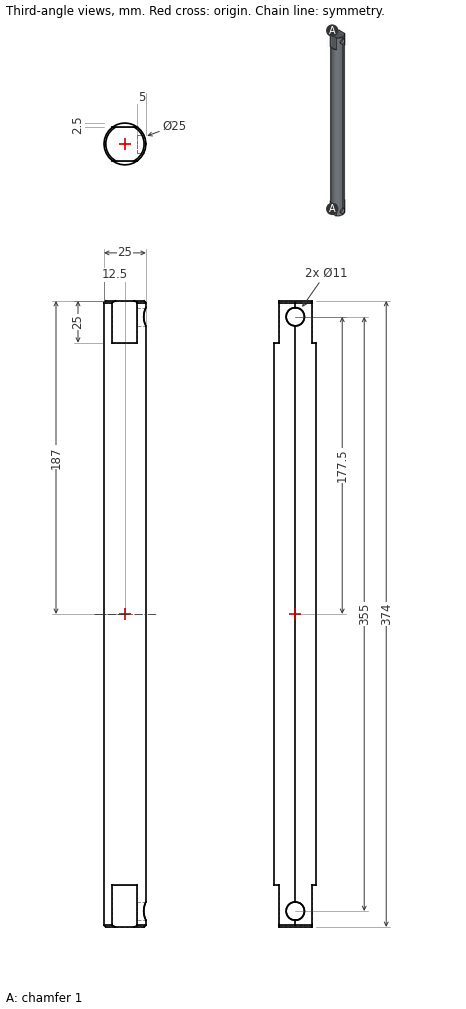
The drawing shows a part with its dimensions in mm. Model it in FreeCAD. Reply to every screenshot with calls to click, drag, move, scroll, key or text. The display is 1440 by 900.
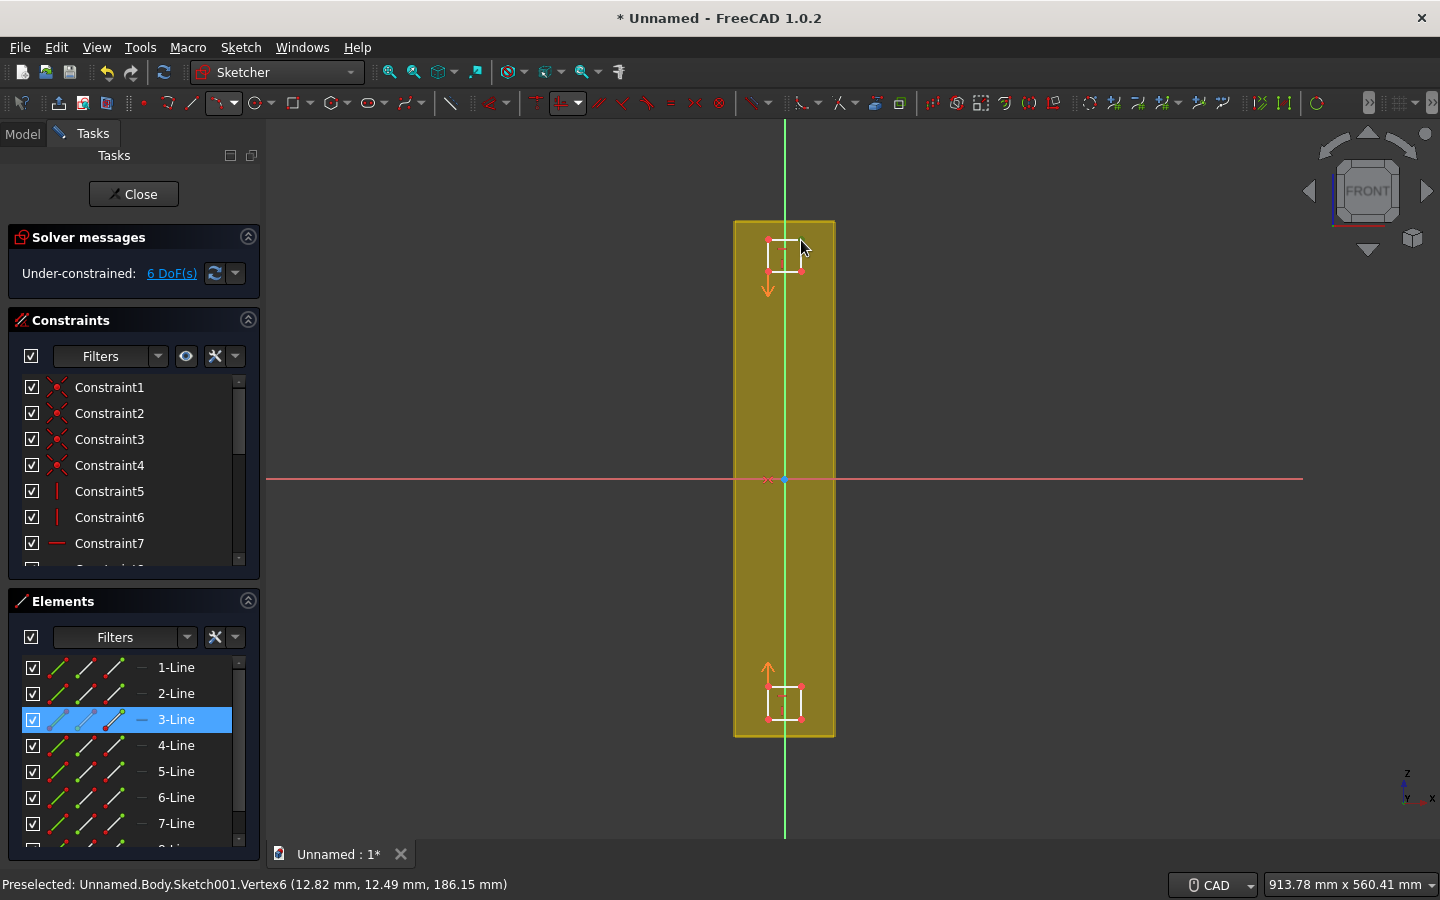
click(801, 720)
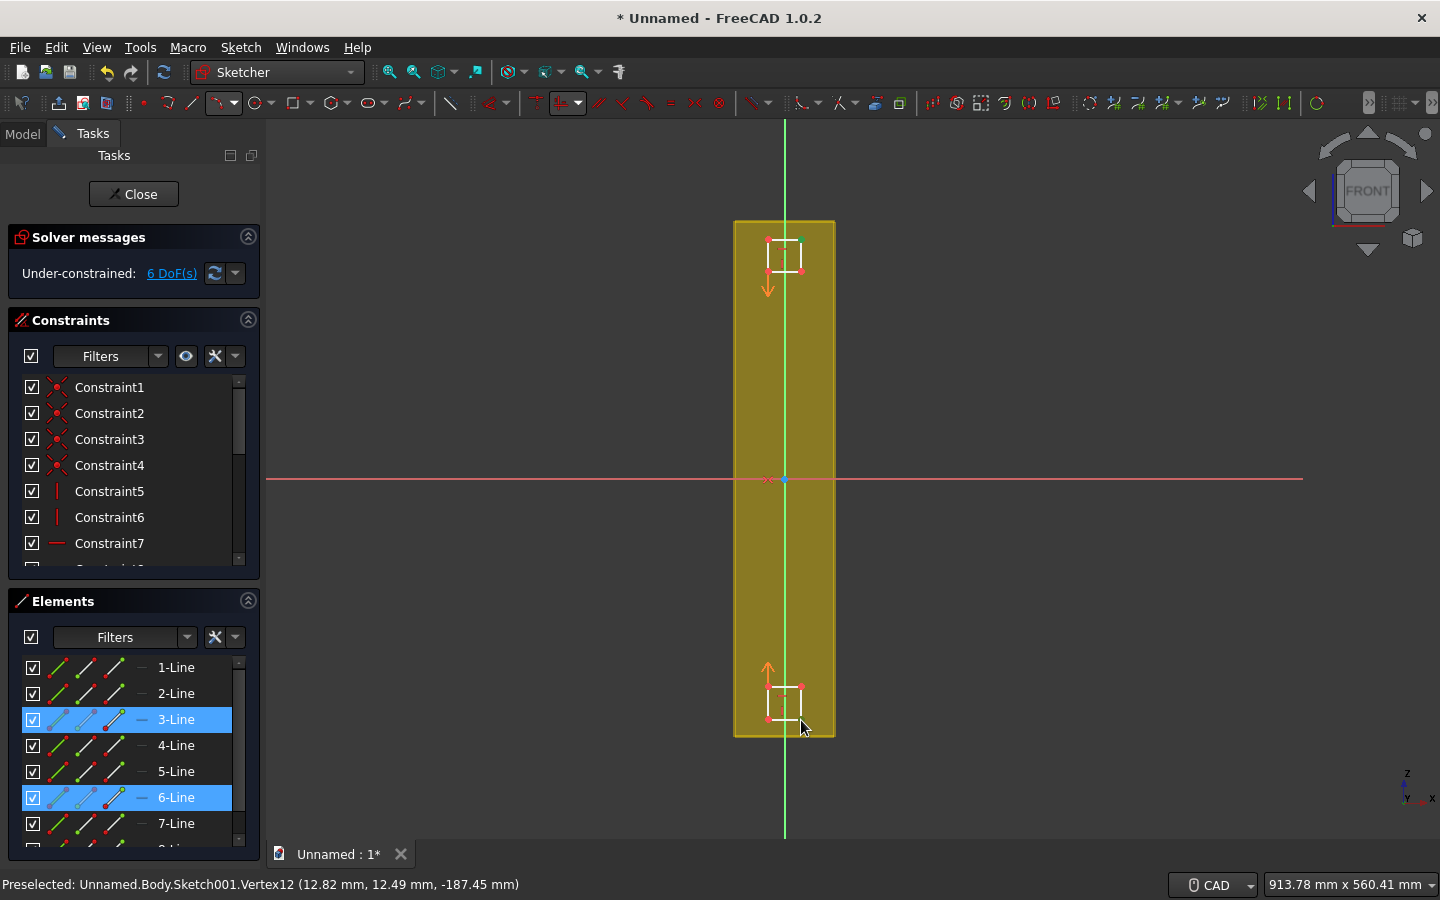
click(364, 479)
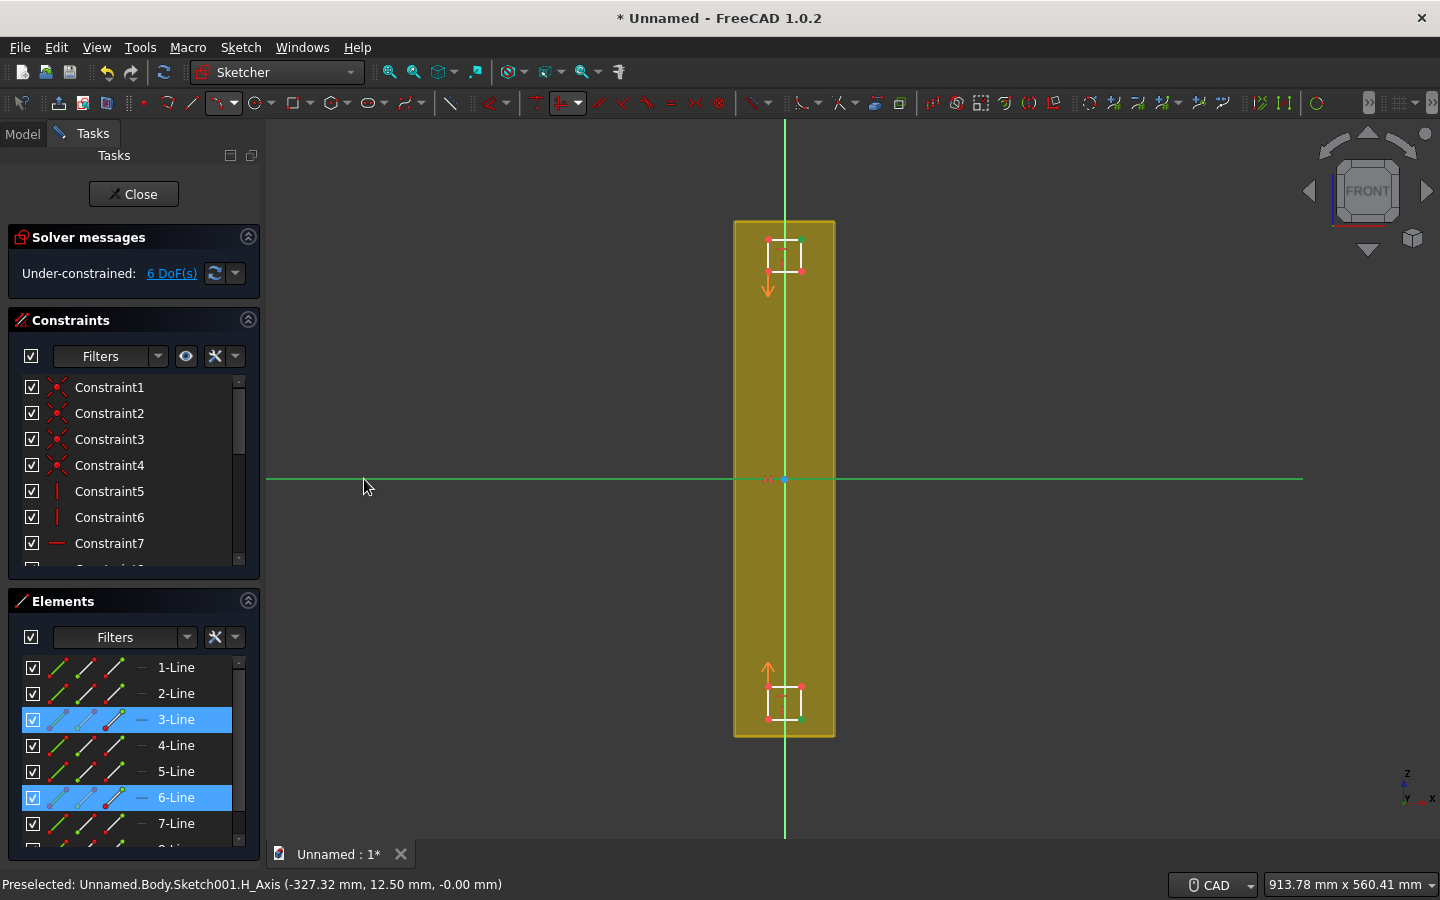
key(s)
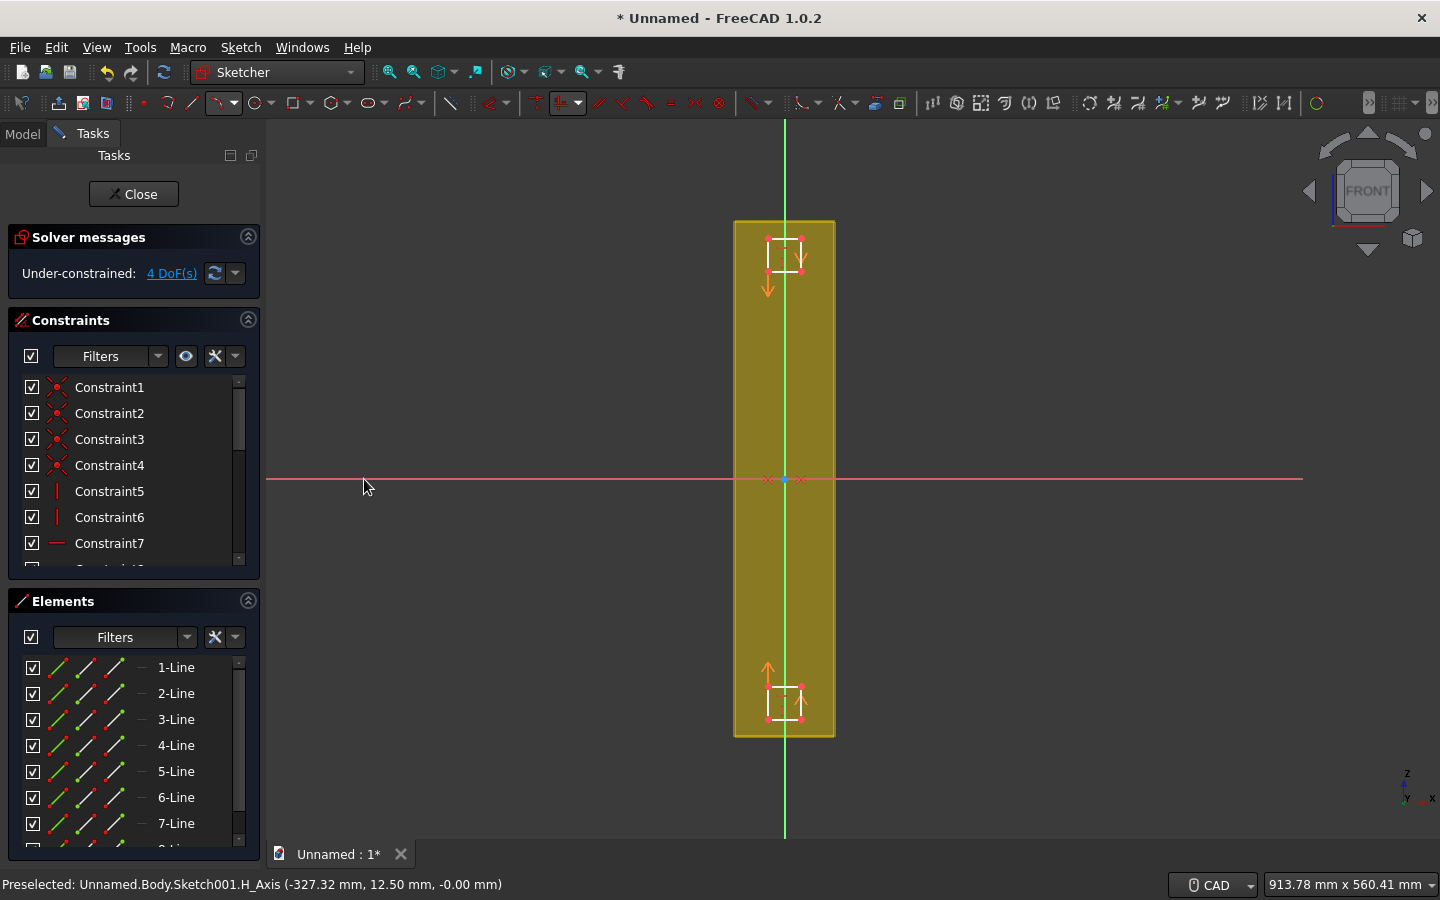
key(d)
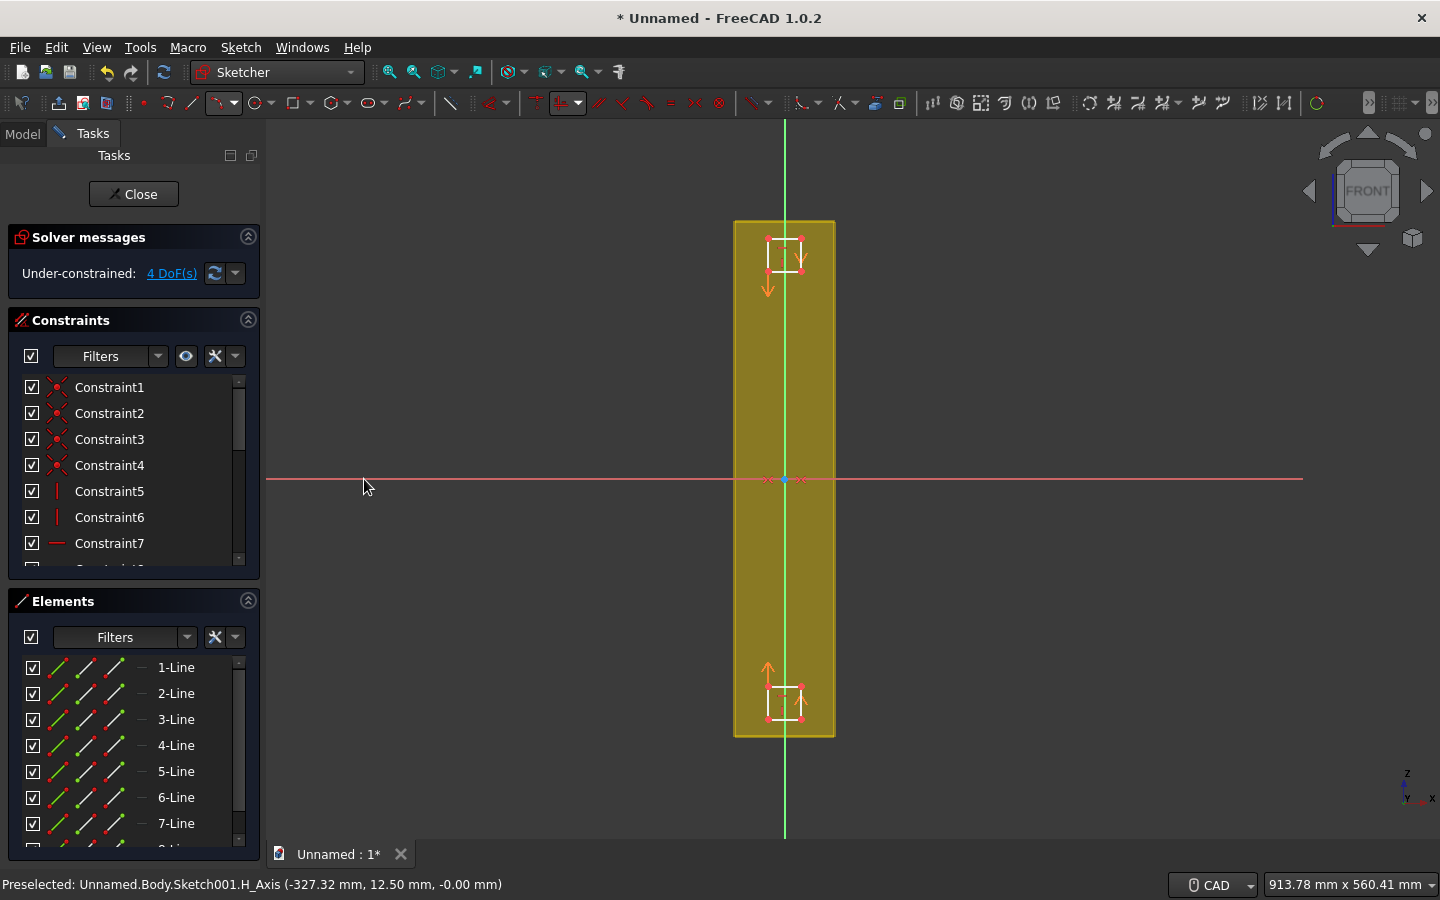
scroll(768, 249, up, 2)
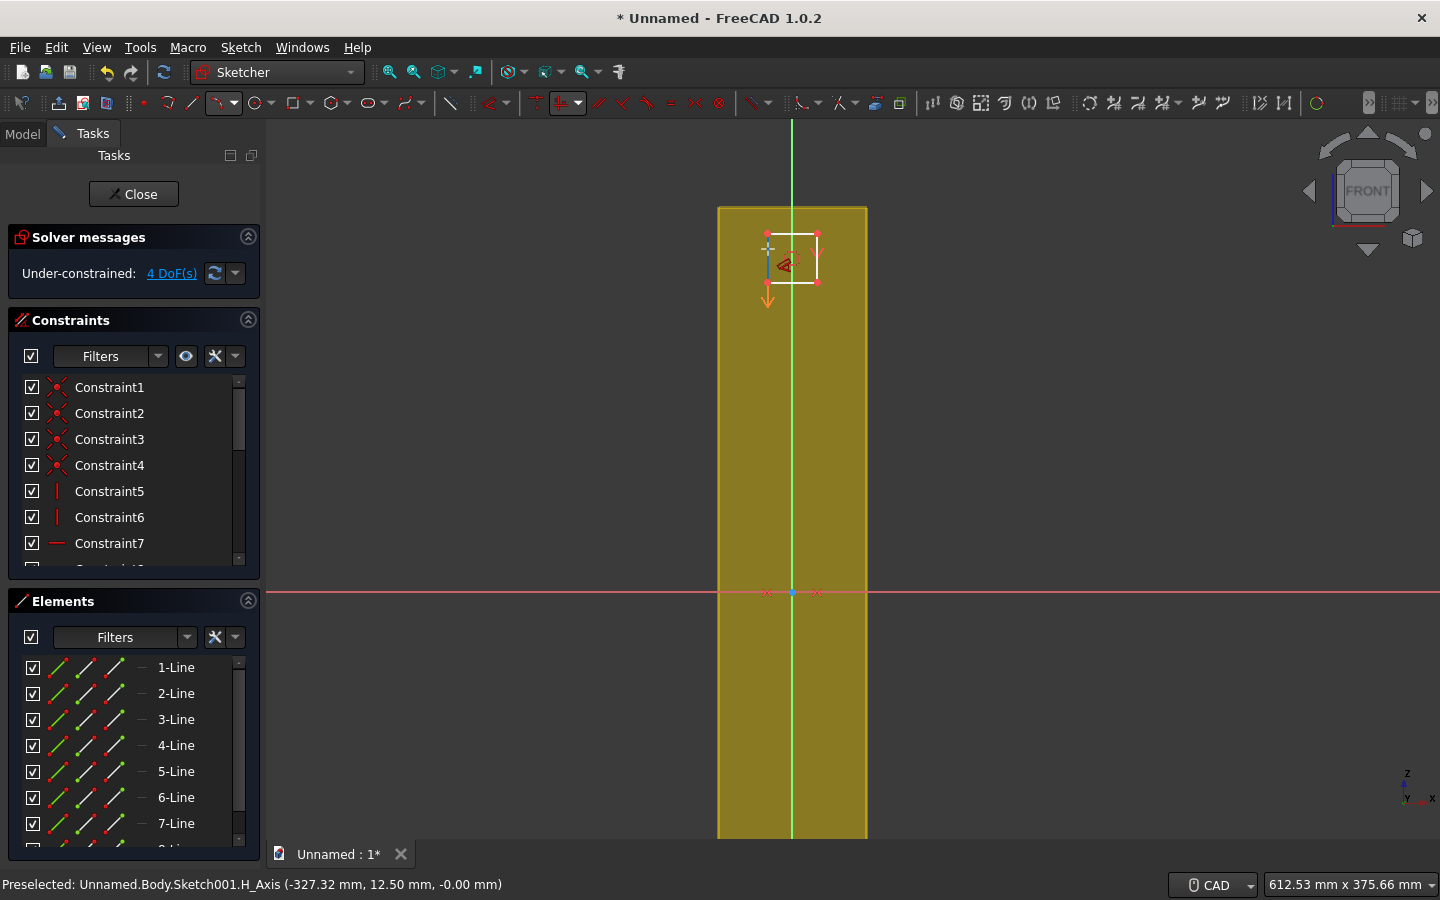
click(768, 248)
click(734, 258)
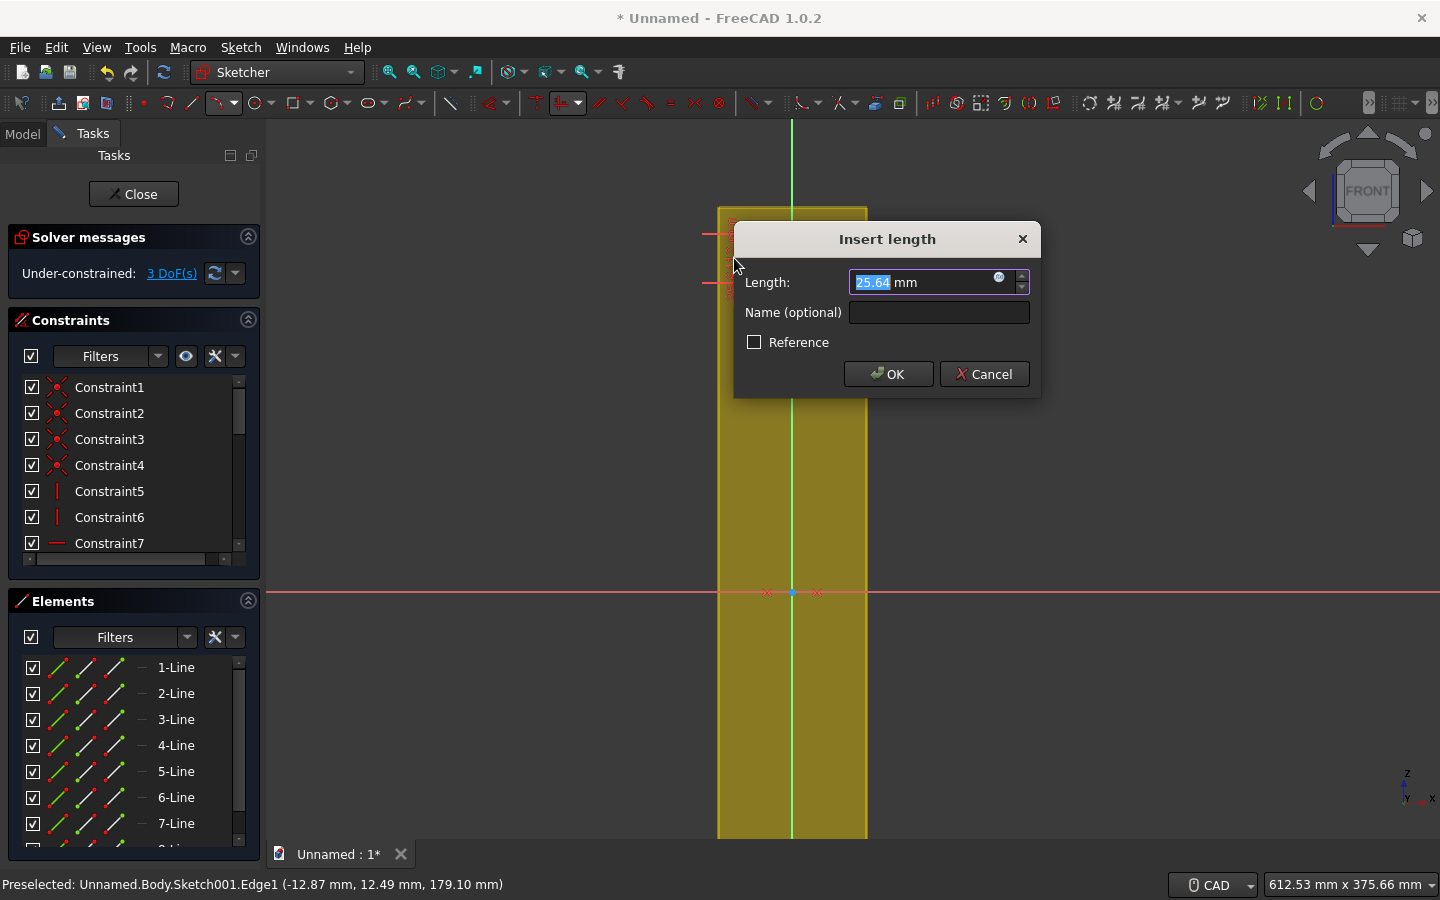
text(25)
key(Return)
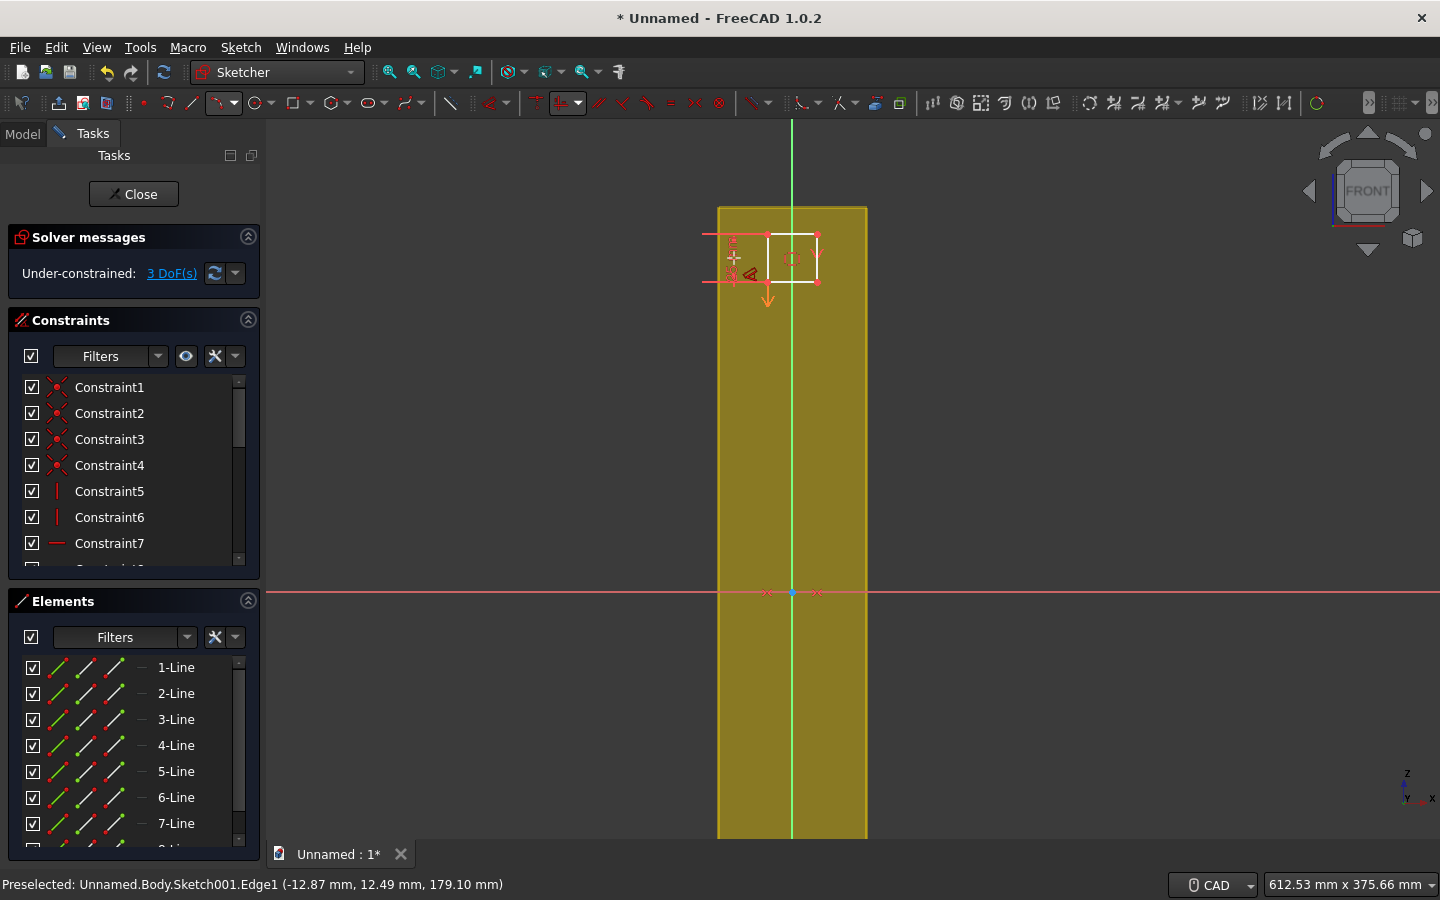
scroll(783, 282, up, 2)